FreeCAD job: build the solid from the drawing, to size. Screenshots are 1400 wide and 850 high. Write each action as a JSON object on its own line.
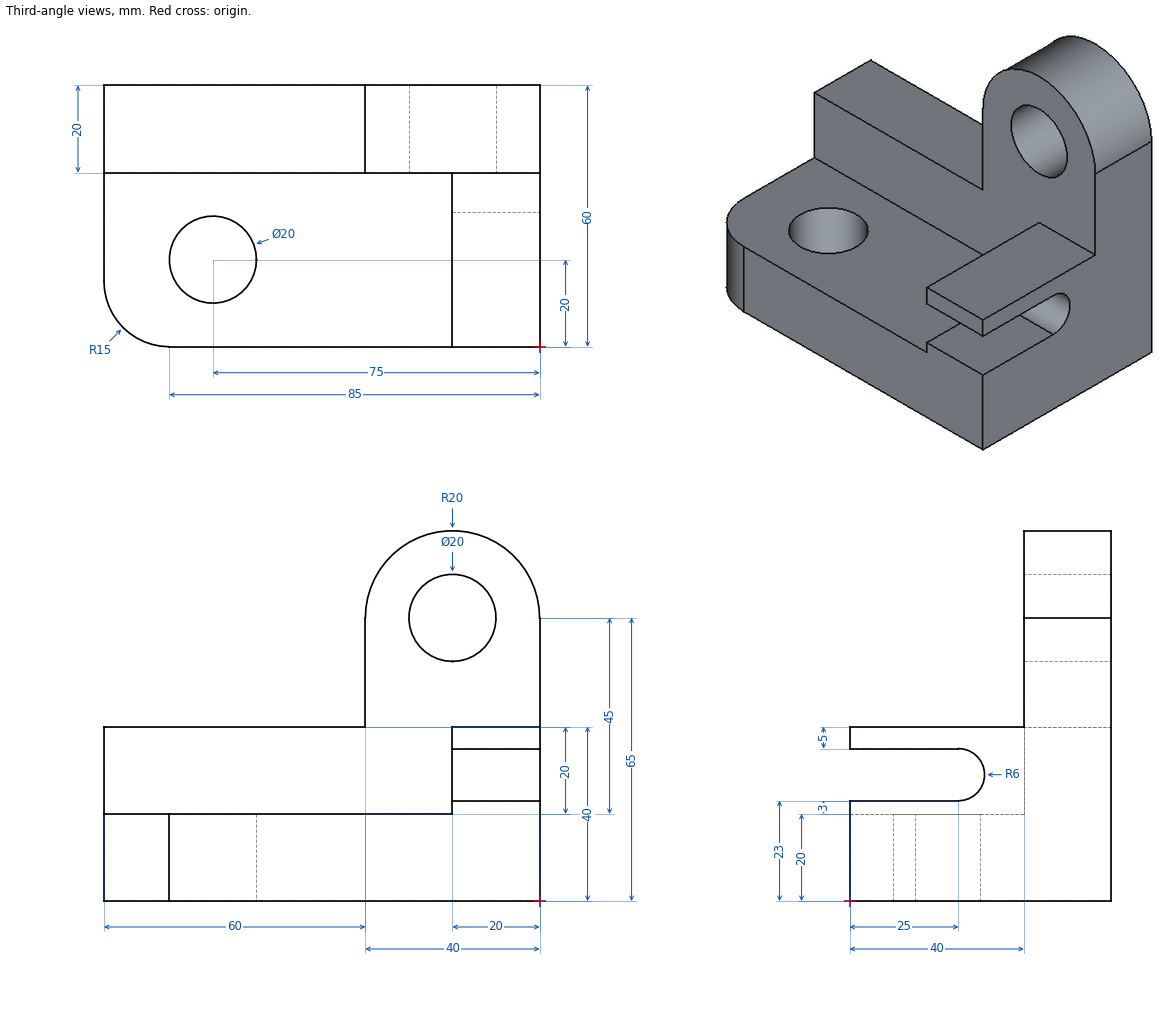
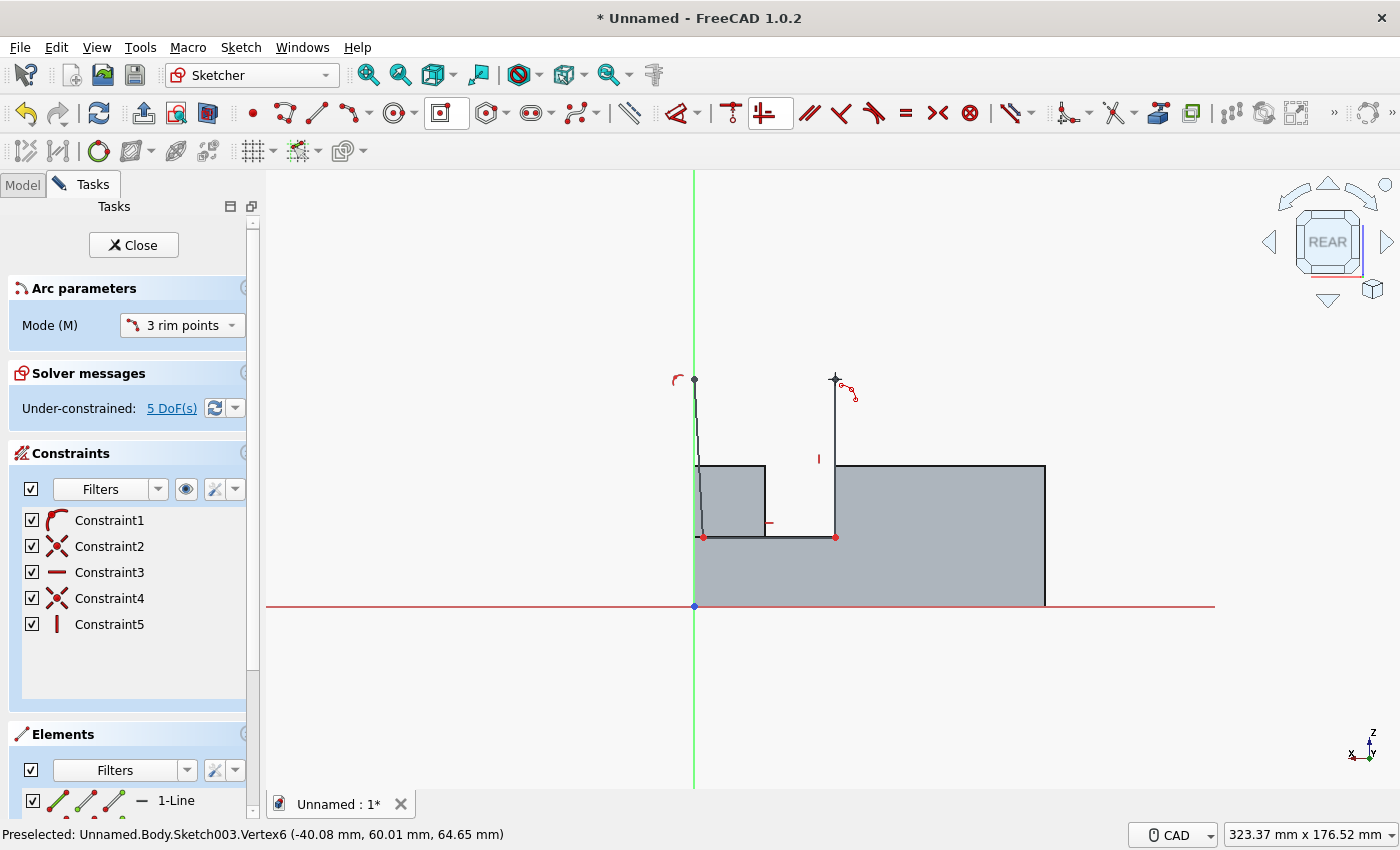
{"action": "left_click", "coordinate": [835, 380]}
{"action": "left_click", "coordinate": [694, 380]}
{"action": "left_click", "coordinate": [765, 309]}
{"action": "key", "text": "Escape"}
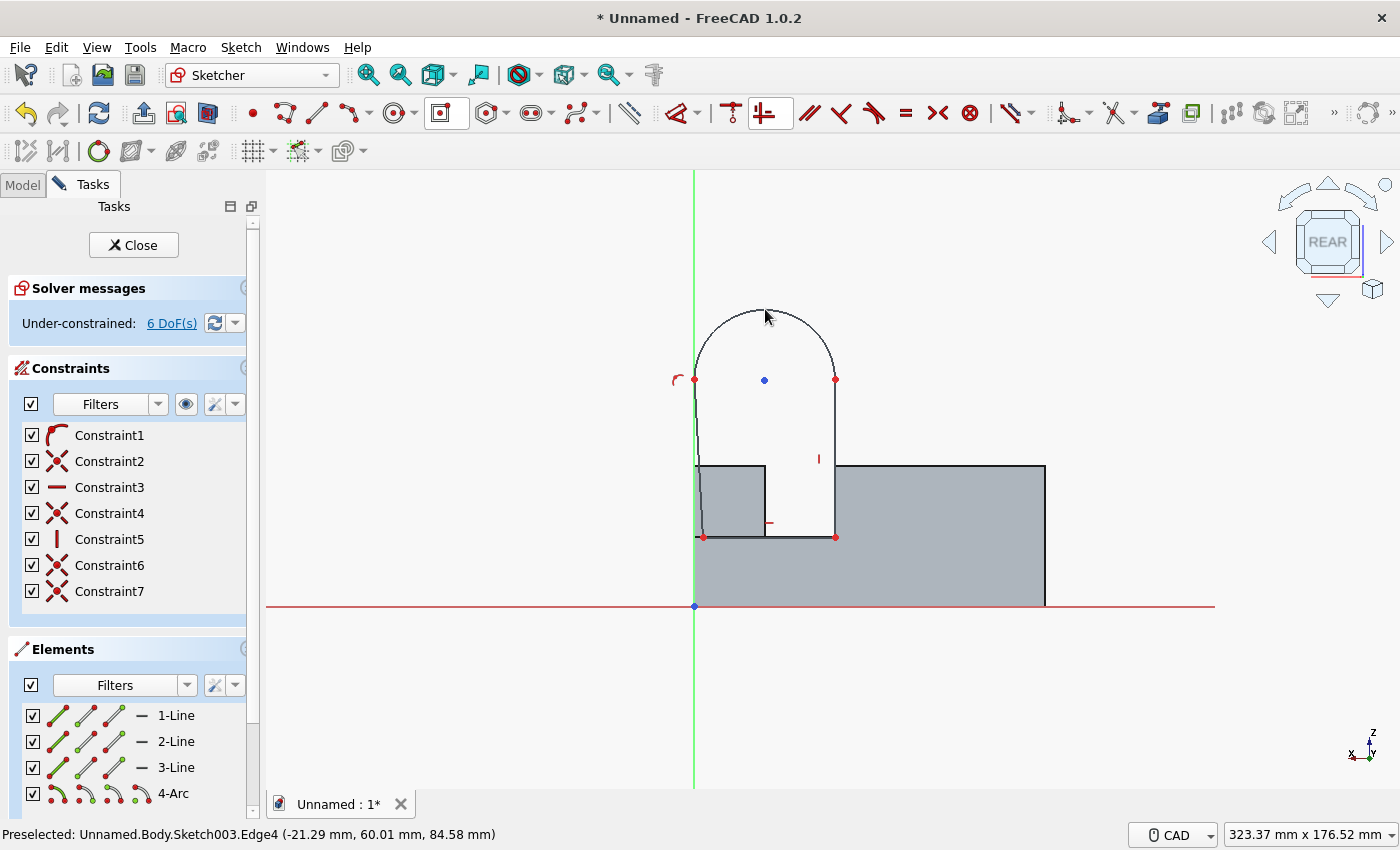
{"action": "left_click", "coordinate": [697, 427]}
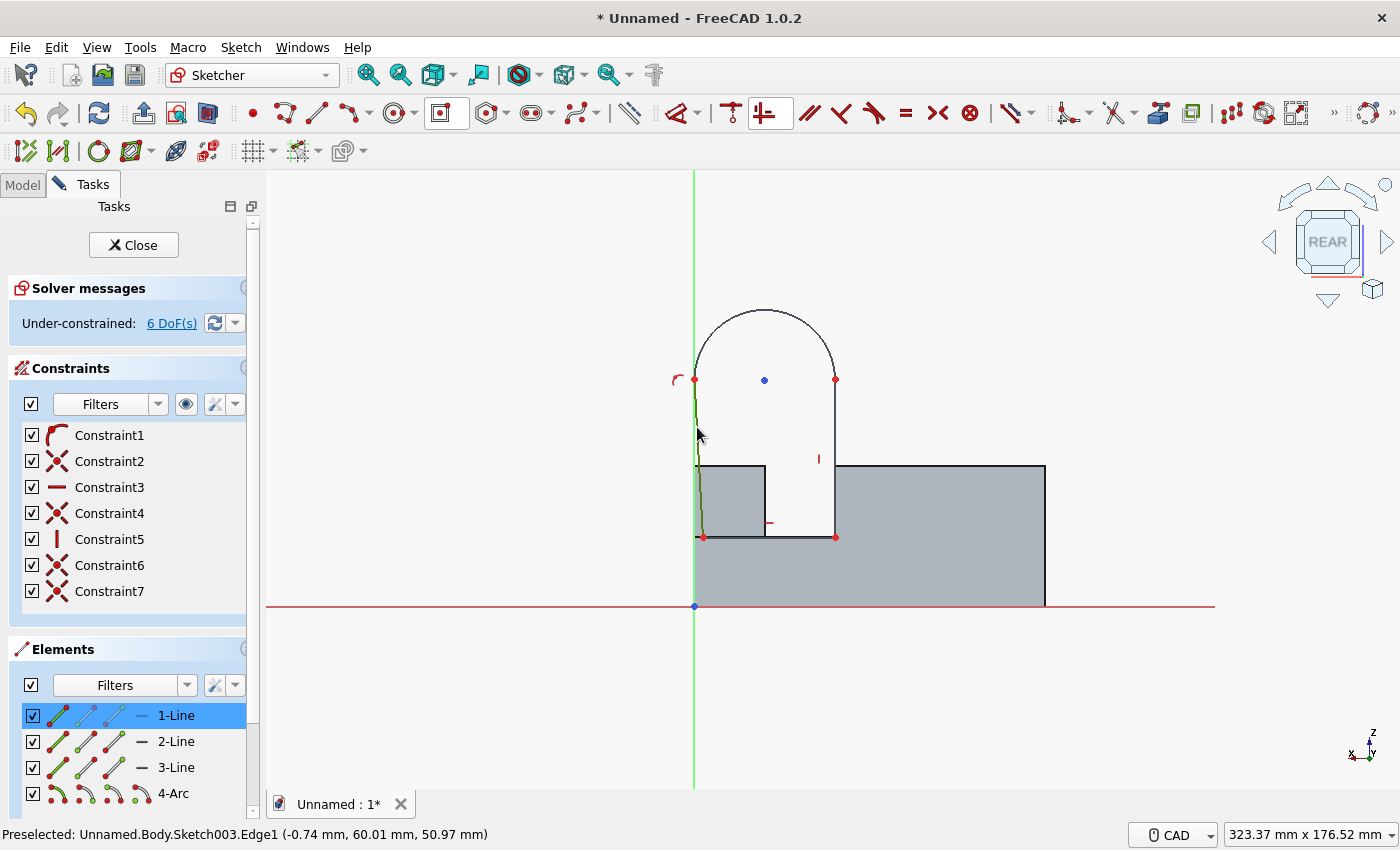
{"action": "left_click", "coordinate": [806, 323]}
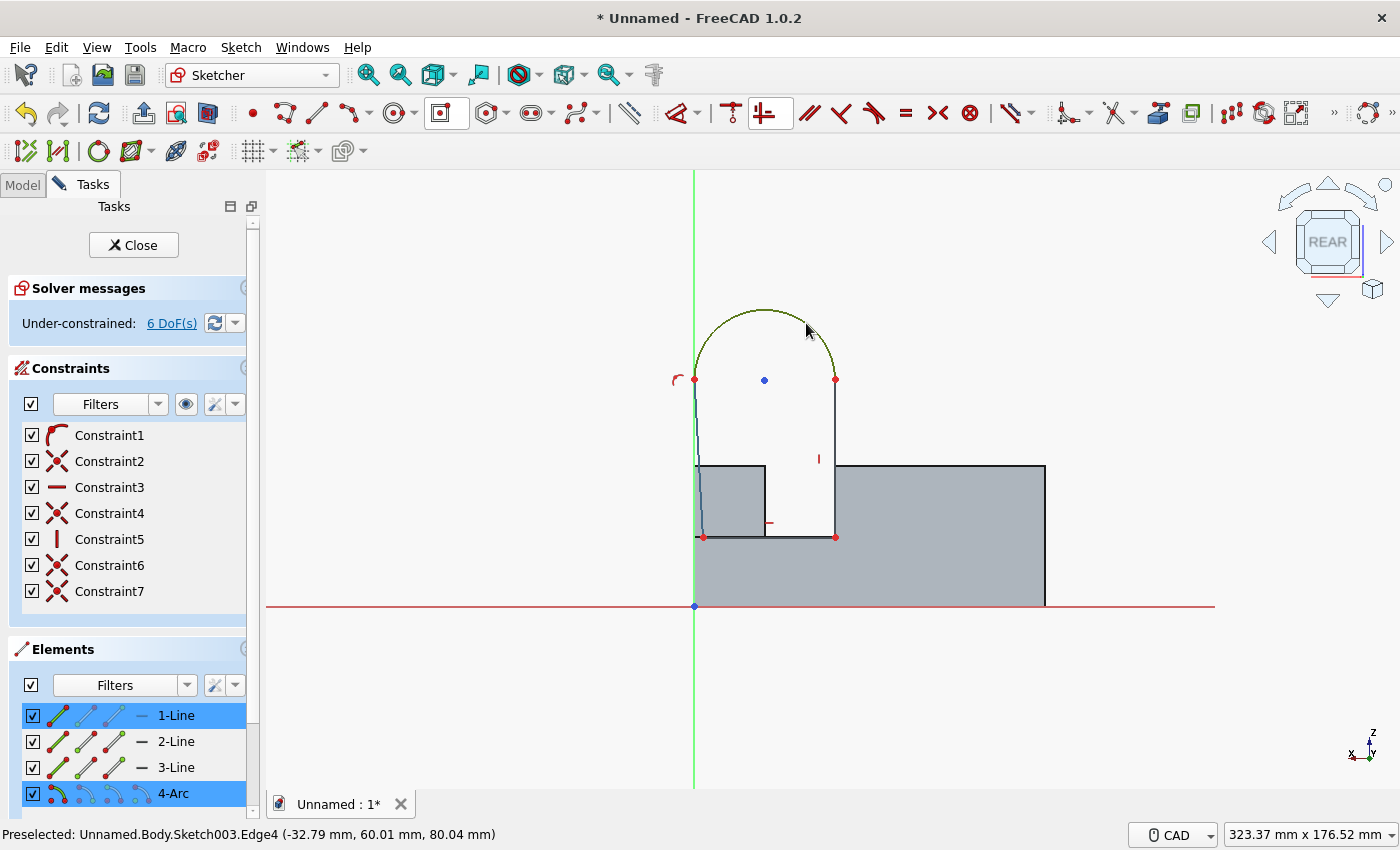
{"action": "left_click", "coordinate": [874, 114]}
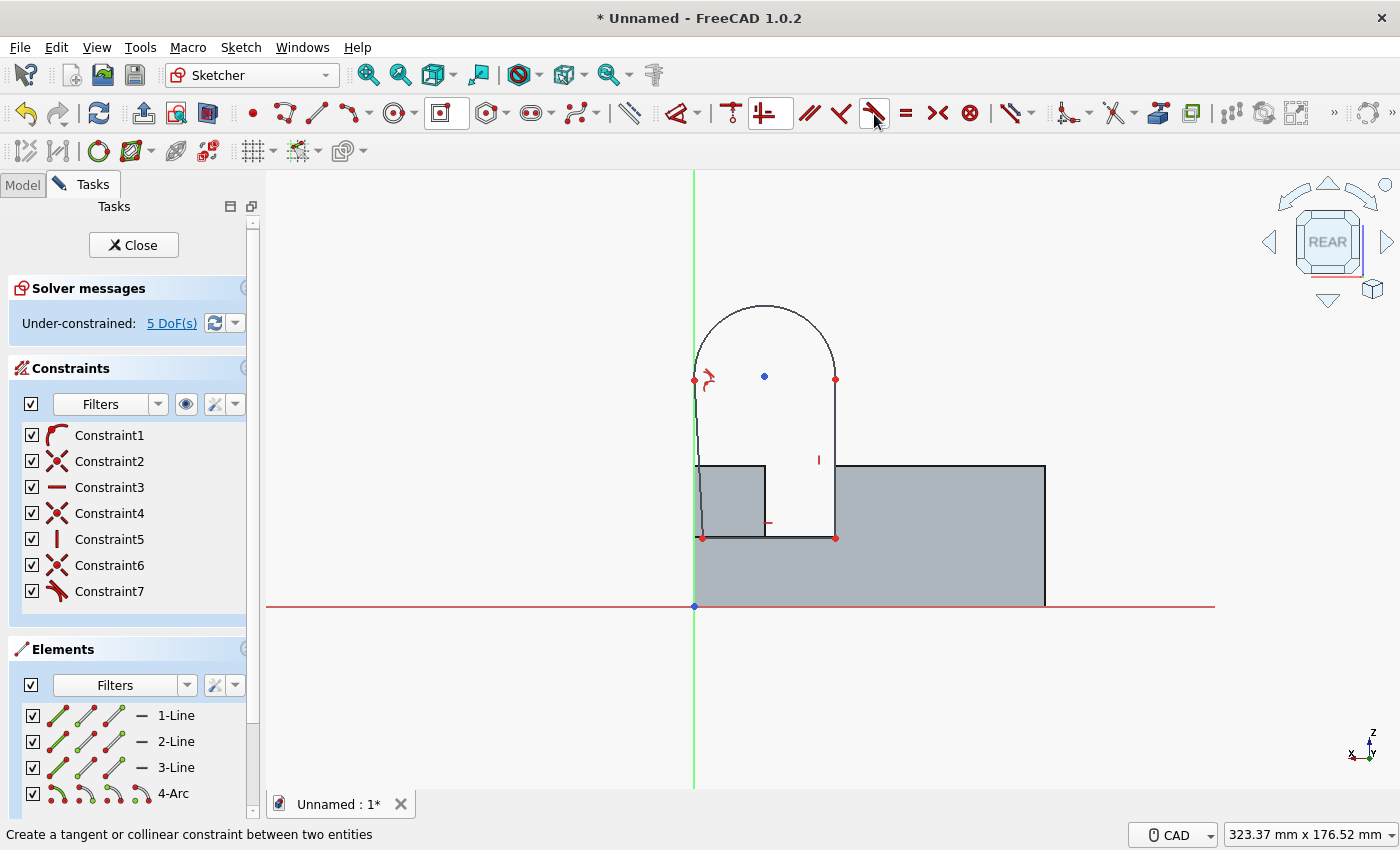
{"action": "left_click", "coordinate": [835, 491]}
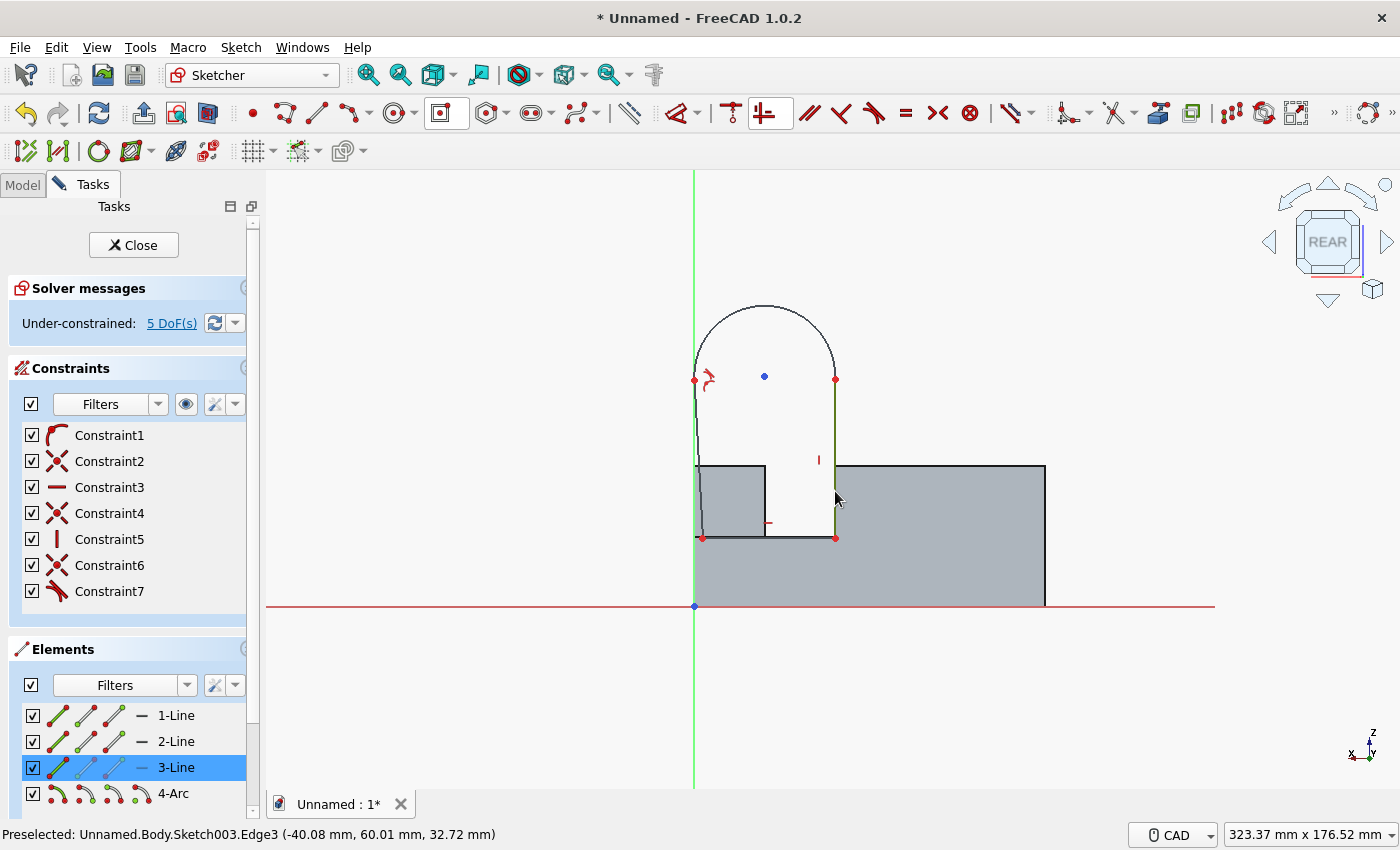
{"action": "left_click", "coordinate": [807, 320]}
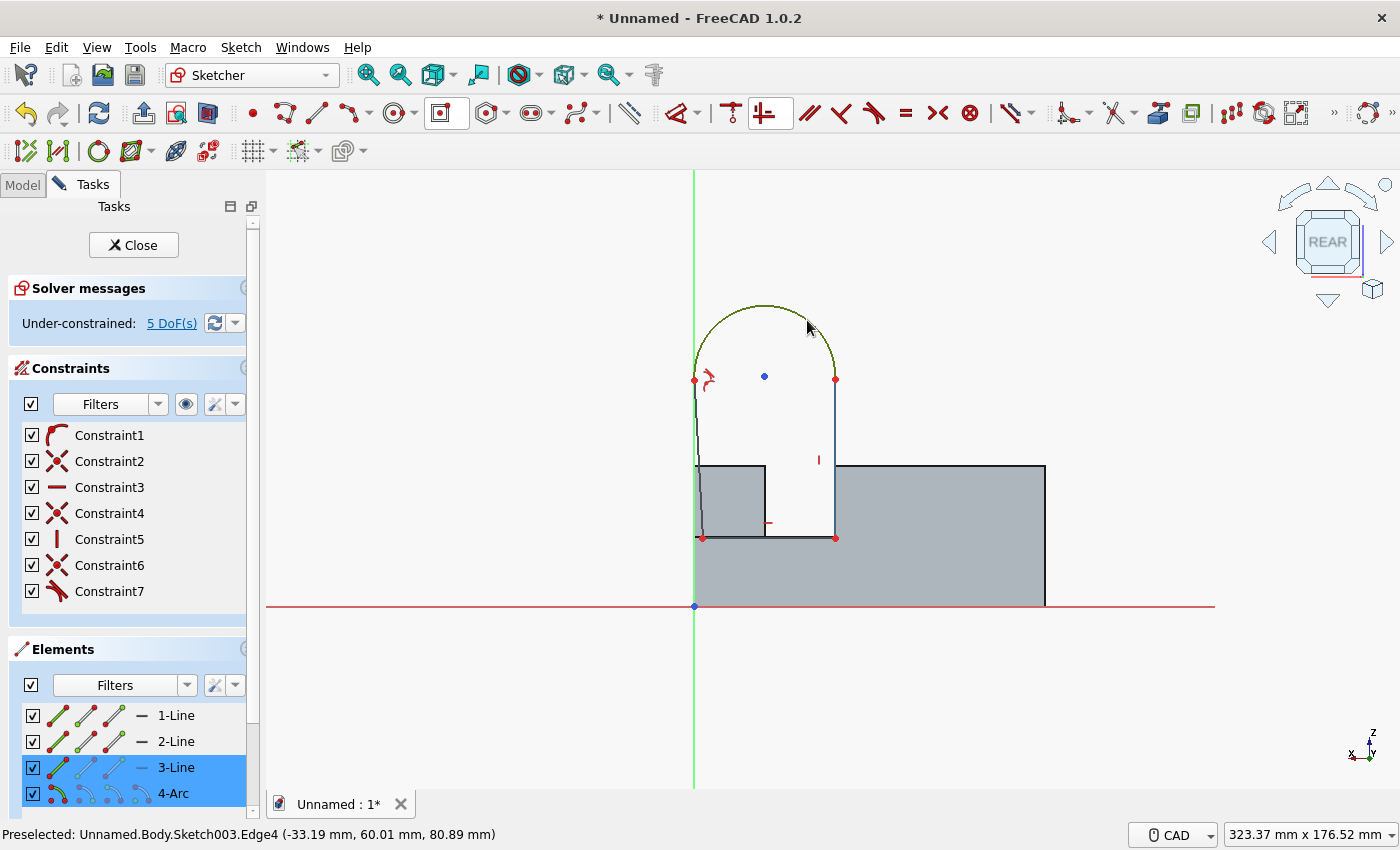
{"action": "left_click", "coordinate": [874, 114]}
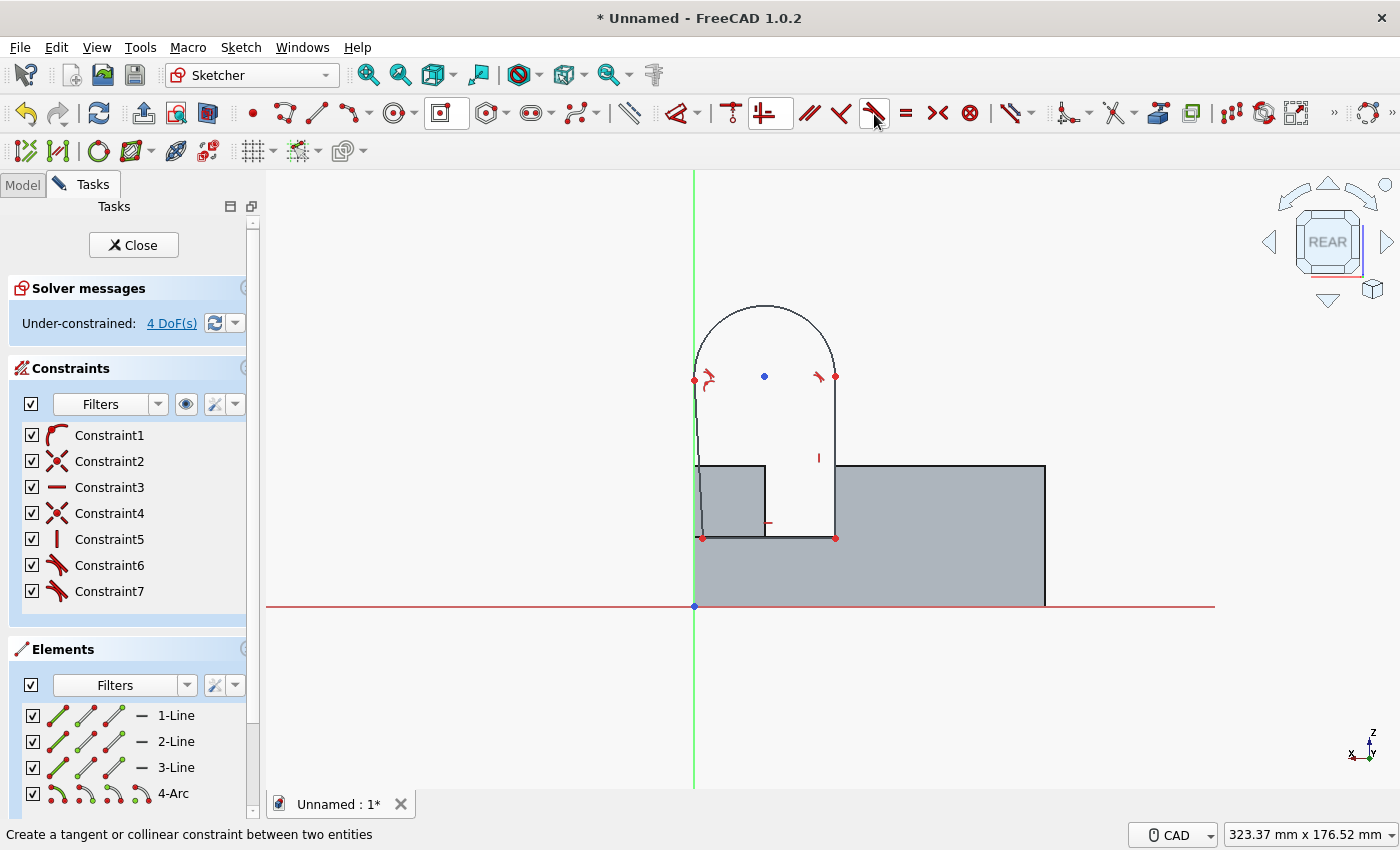
{"action": "left_click", "coordinate": [697, 427]}